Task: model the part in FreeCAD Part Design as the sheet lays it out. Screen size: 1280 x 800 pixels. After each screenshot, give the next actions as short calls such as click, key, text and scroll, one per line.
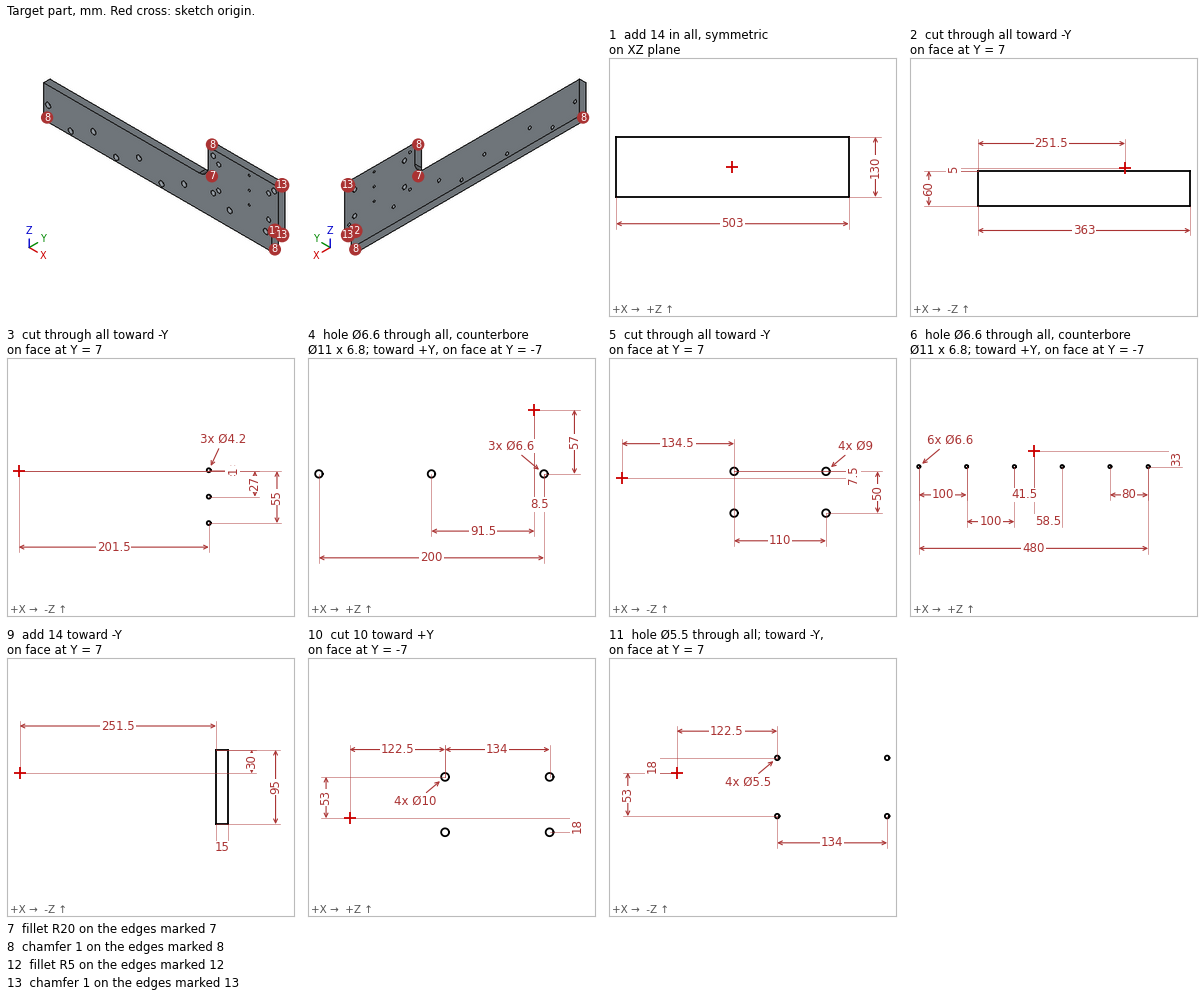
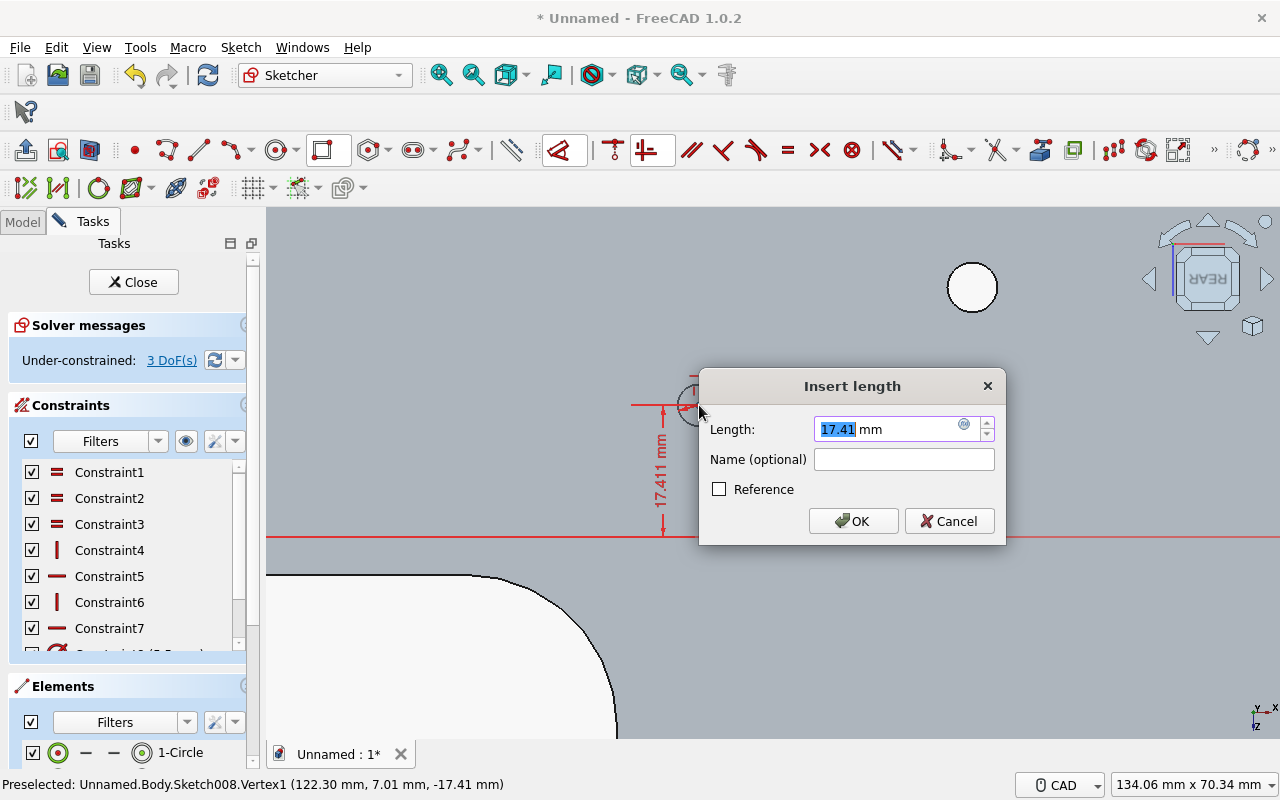
text(18)
key(Return)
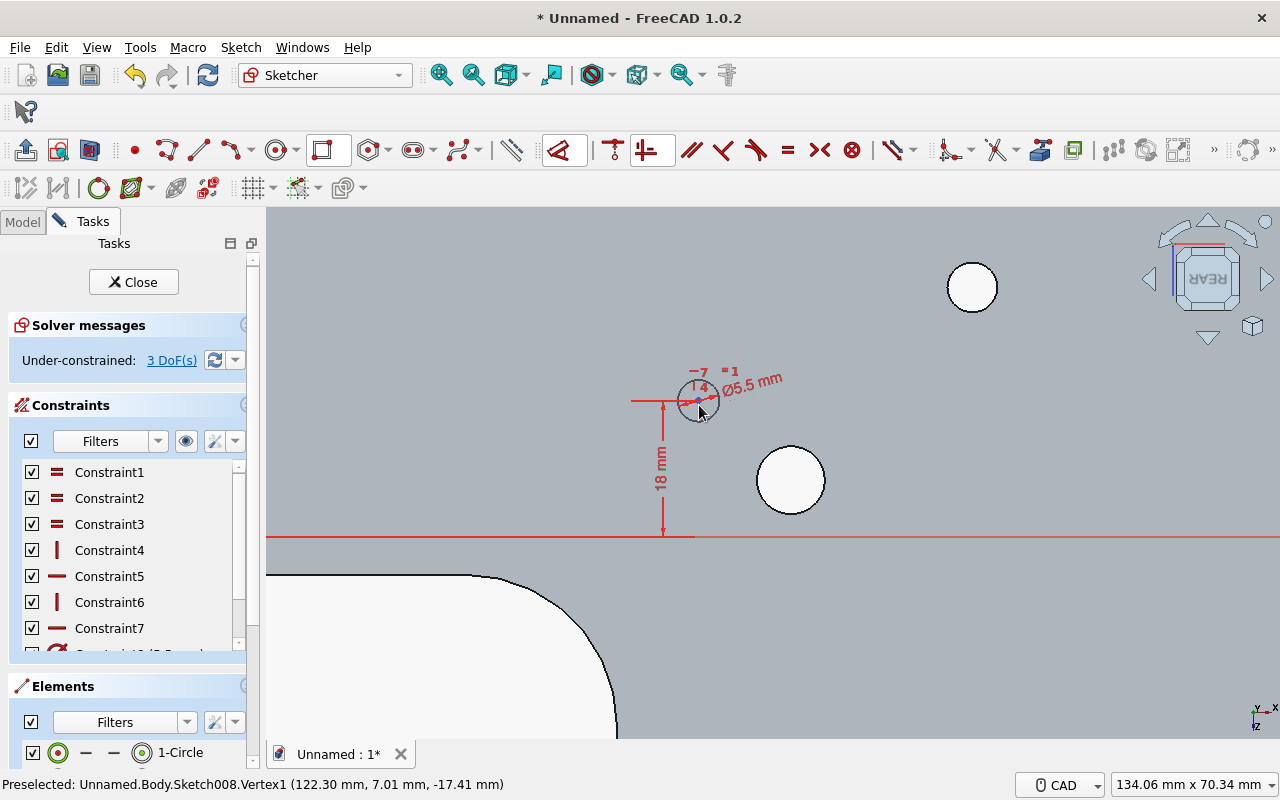
scroll(683, 388, down, 6)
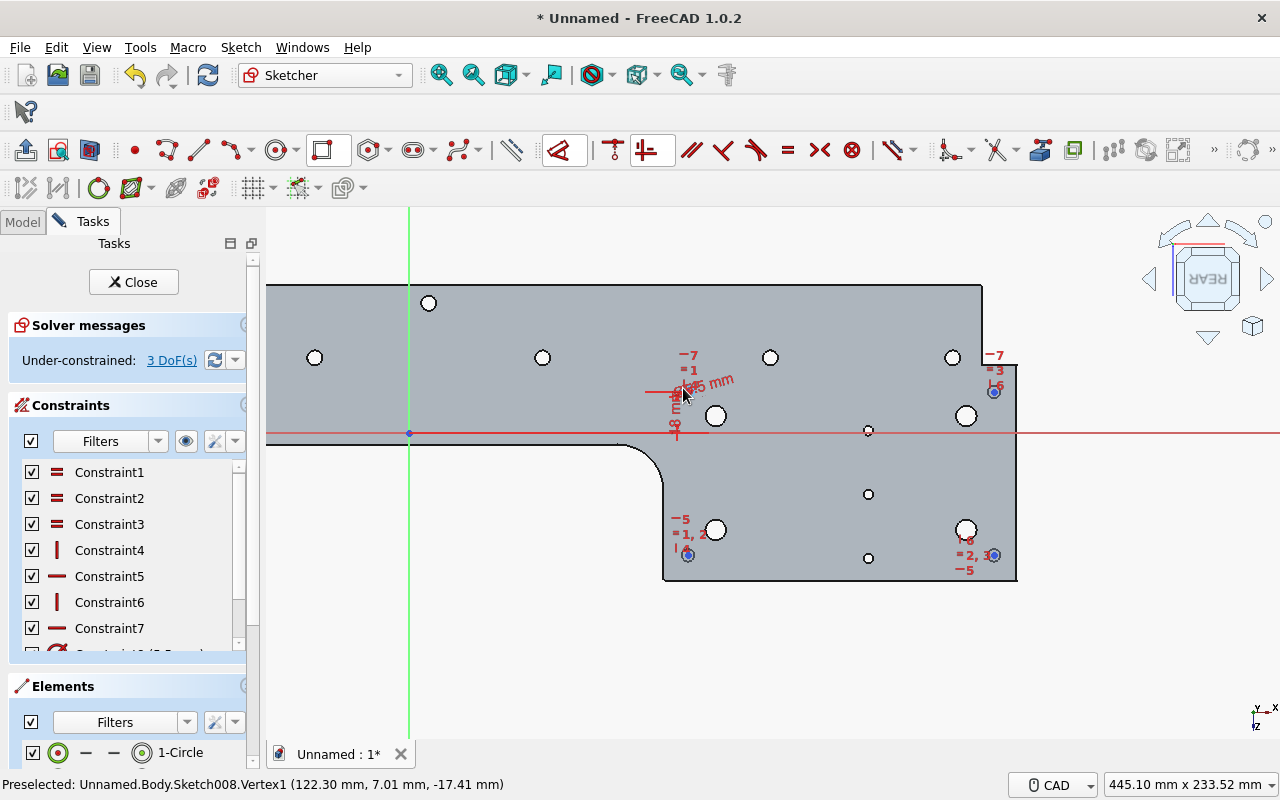
click(688, 555)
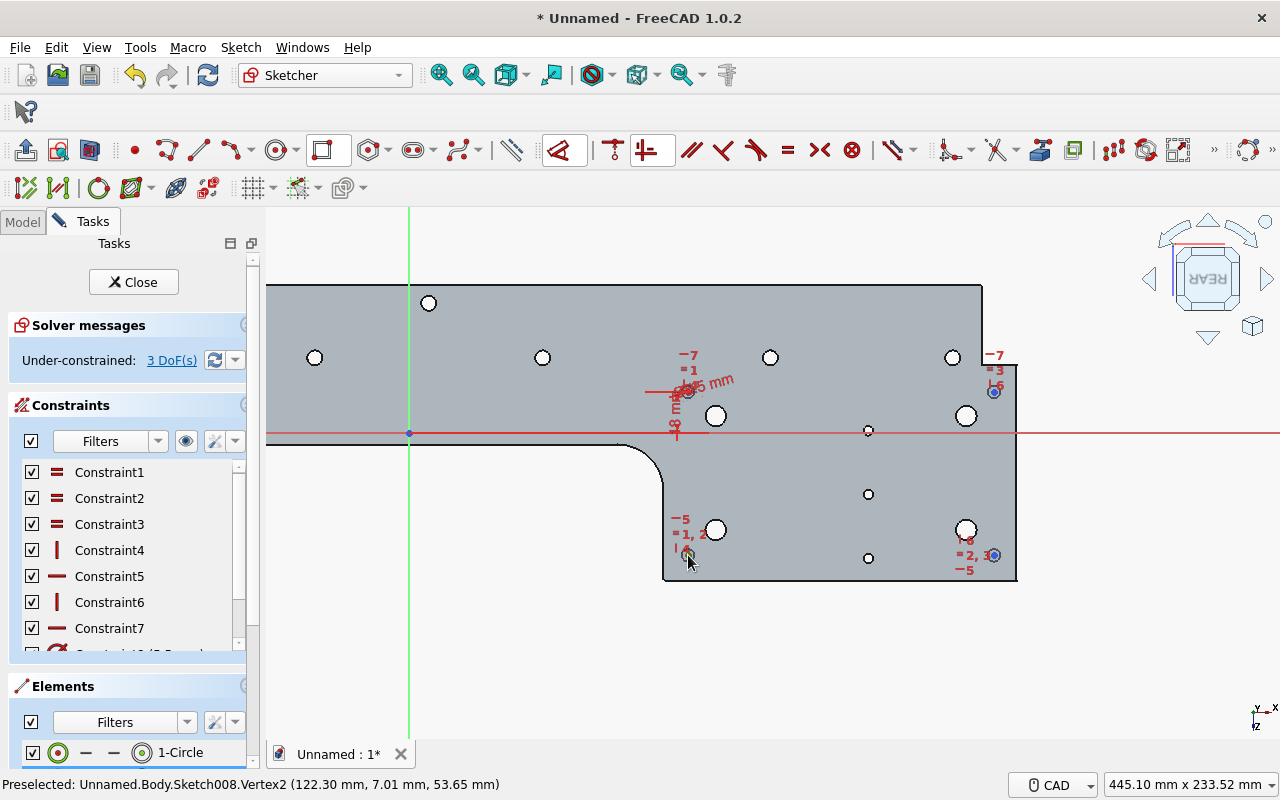
key(i)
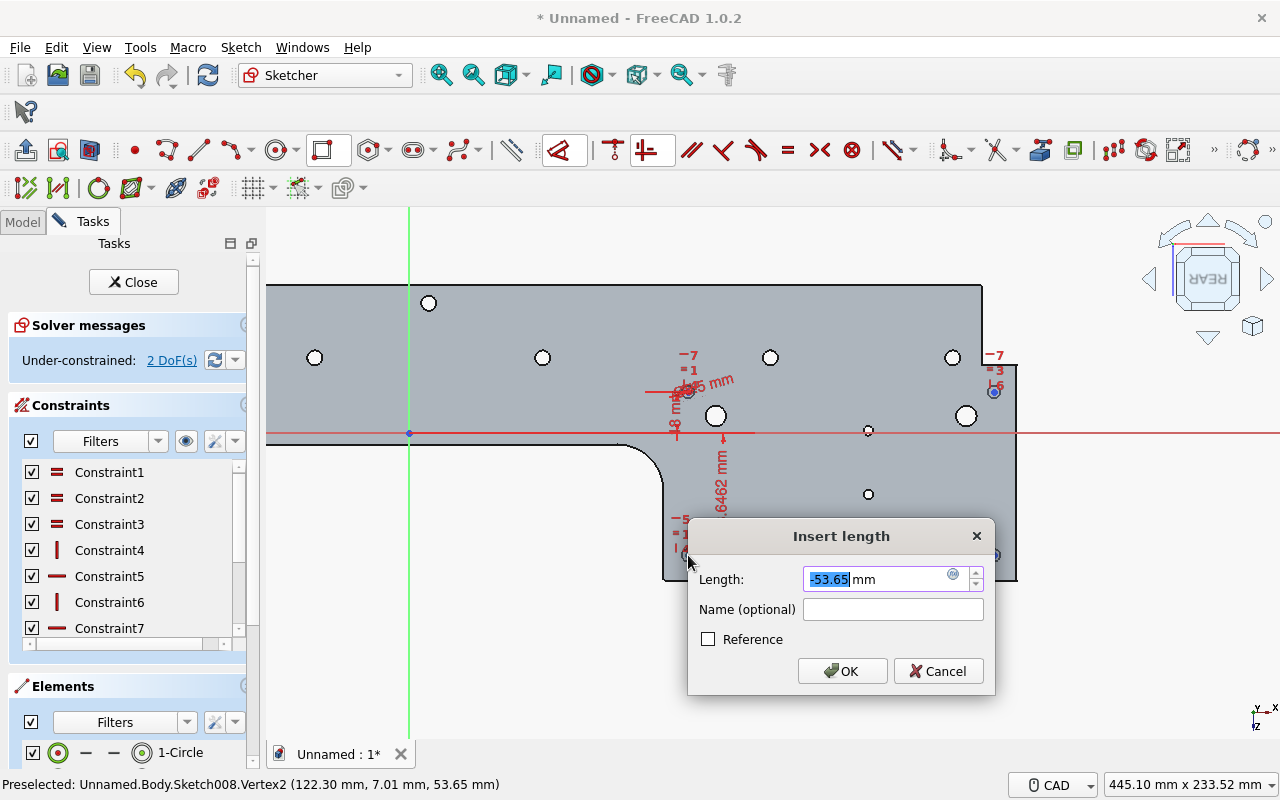
text(-53)
key(Return)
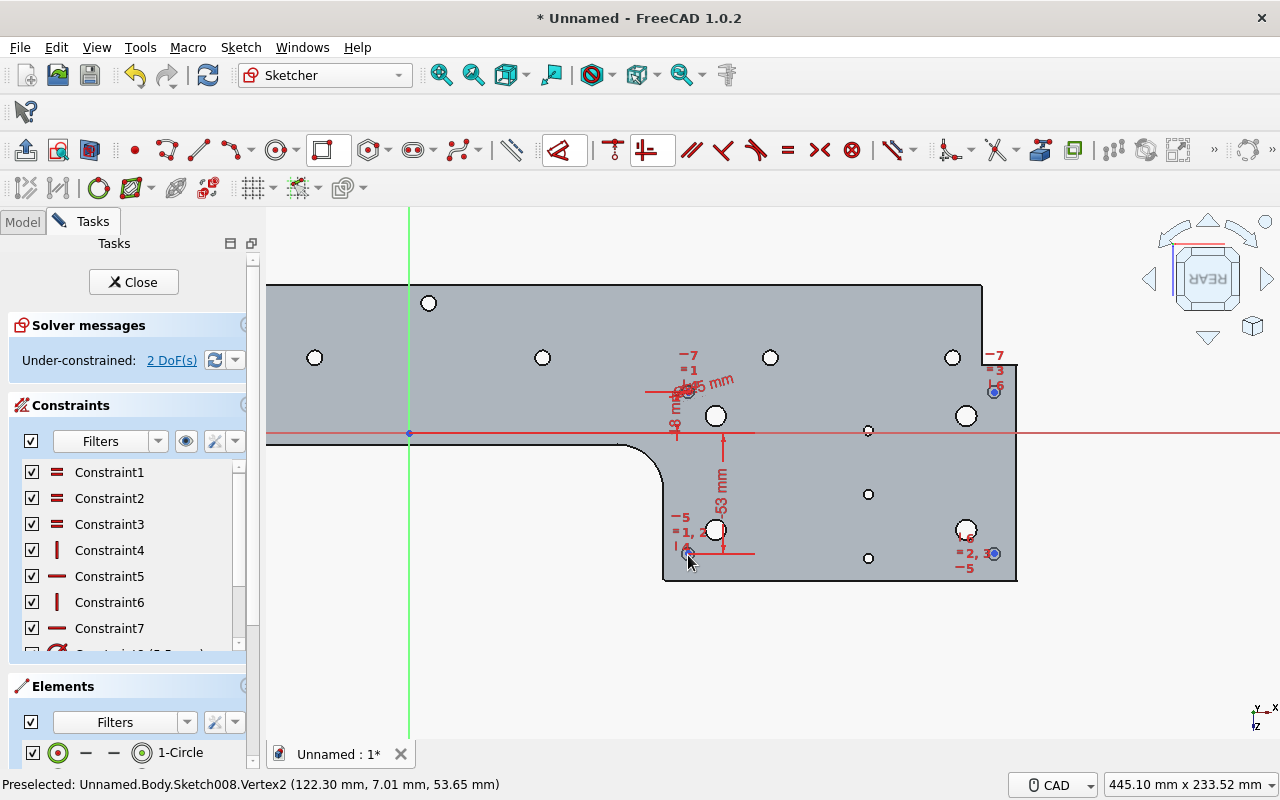
click(688, 554)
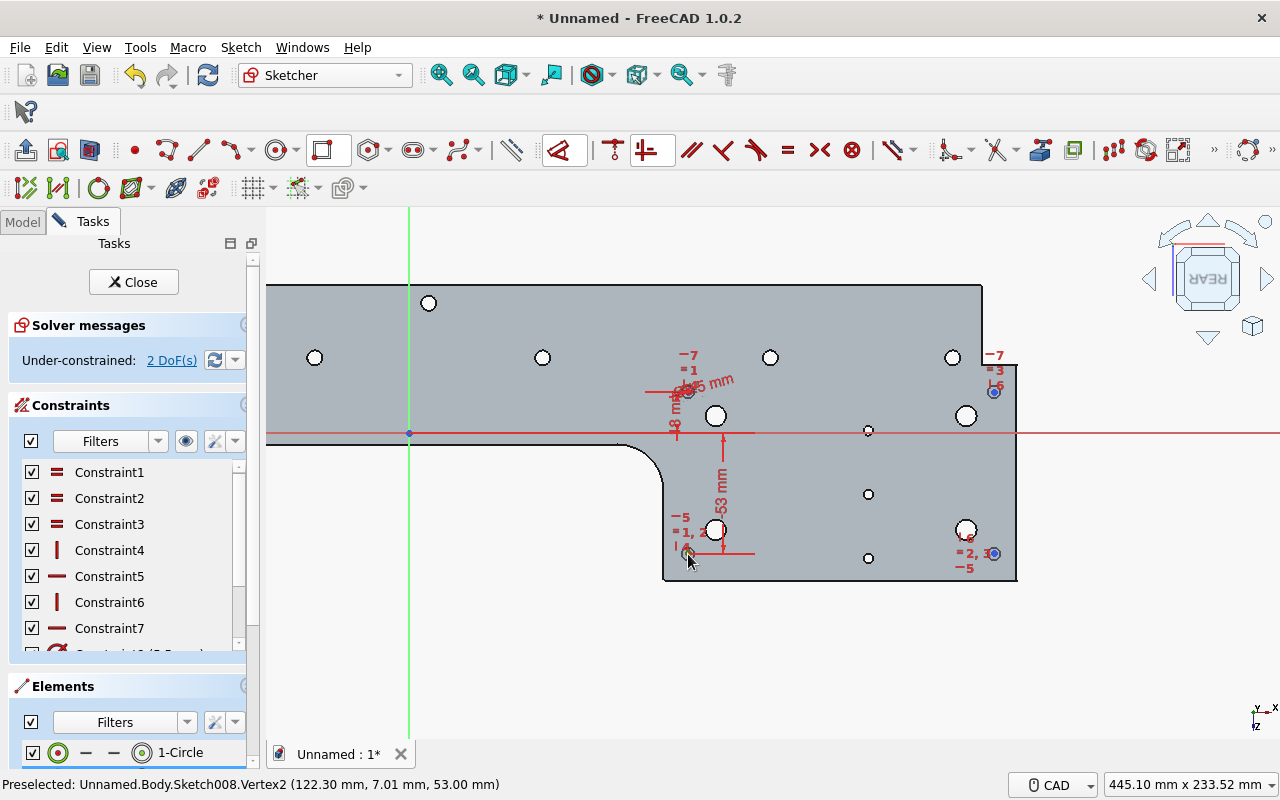
click(994, 554)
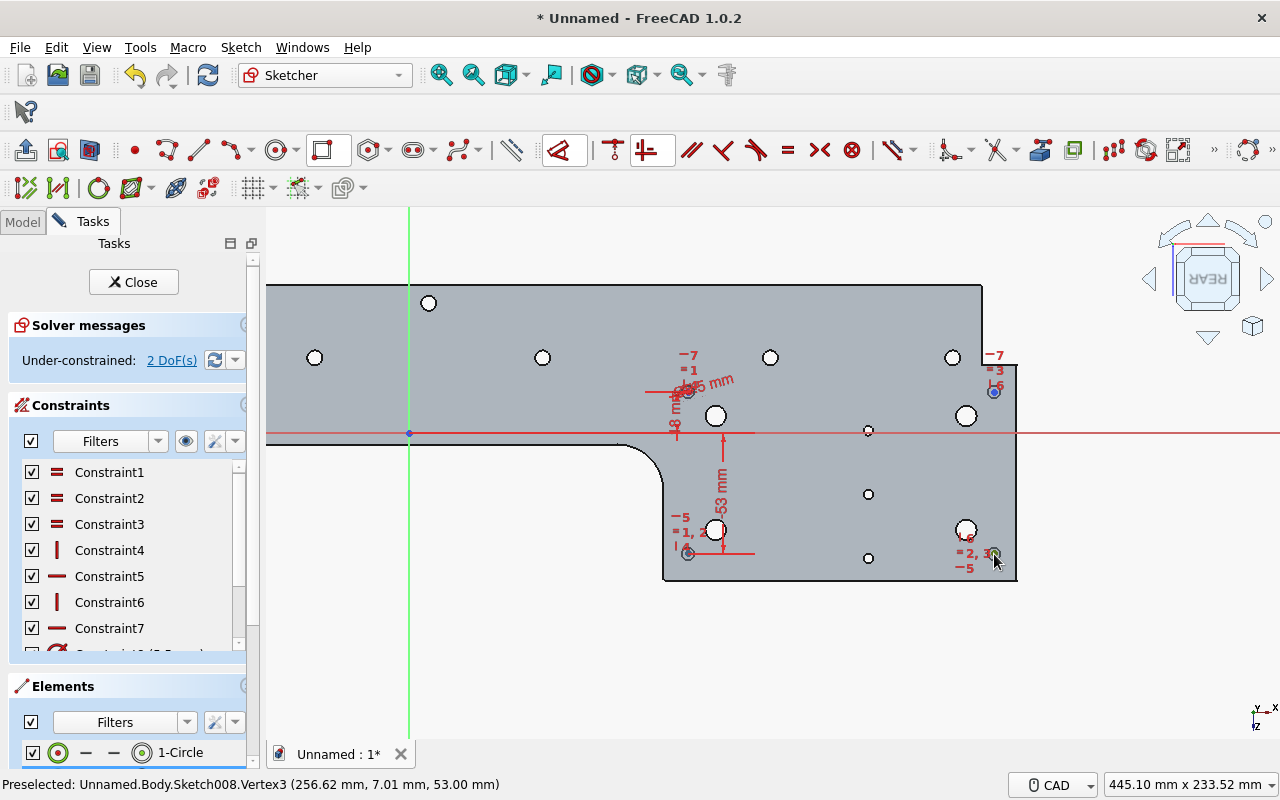
key(l)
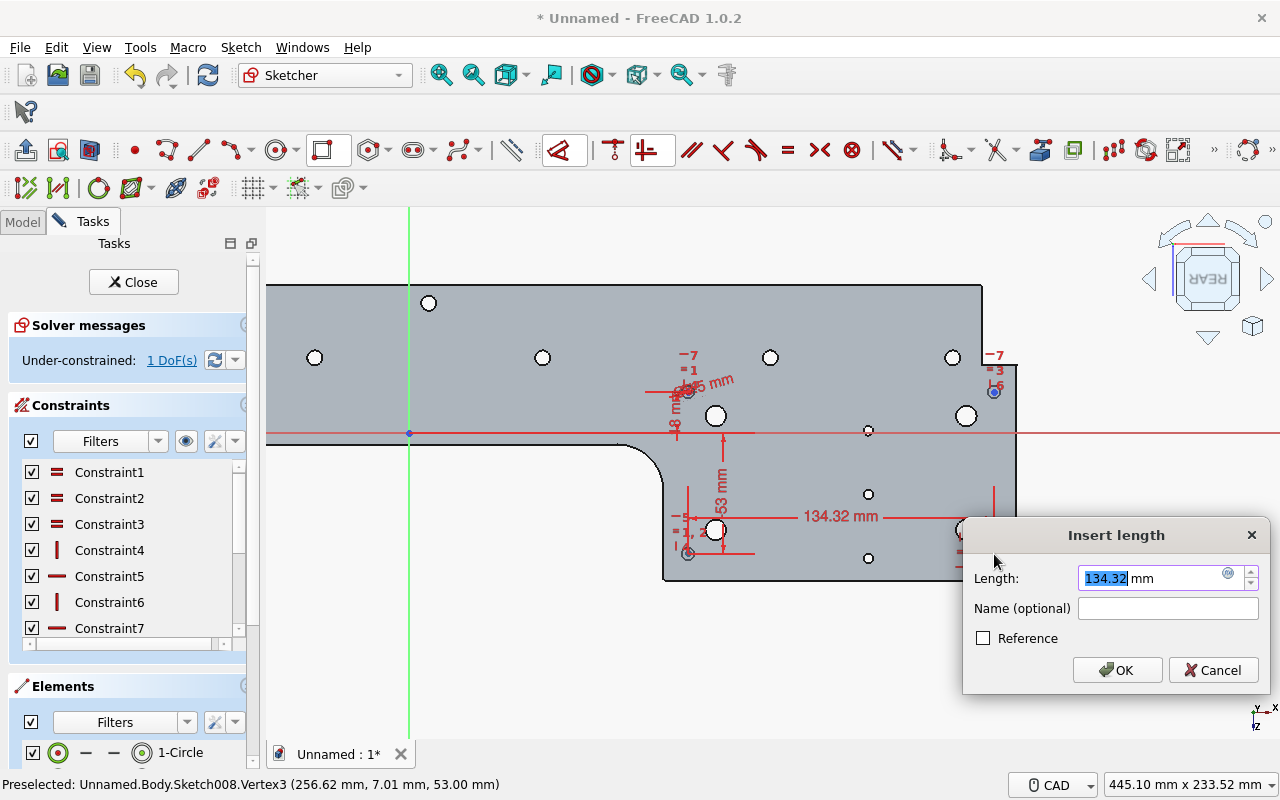
text(134)
key(Return)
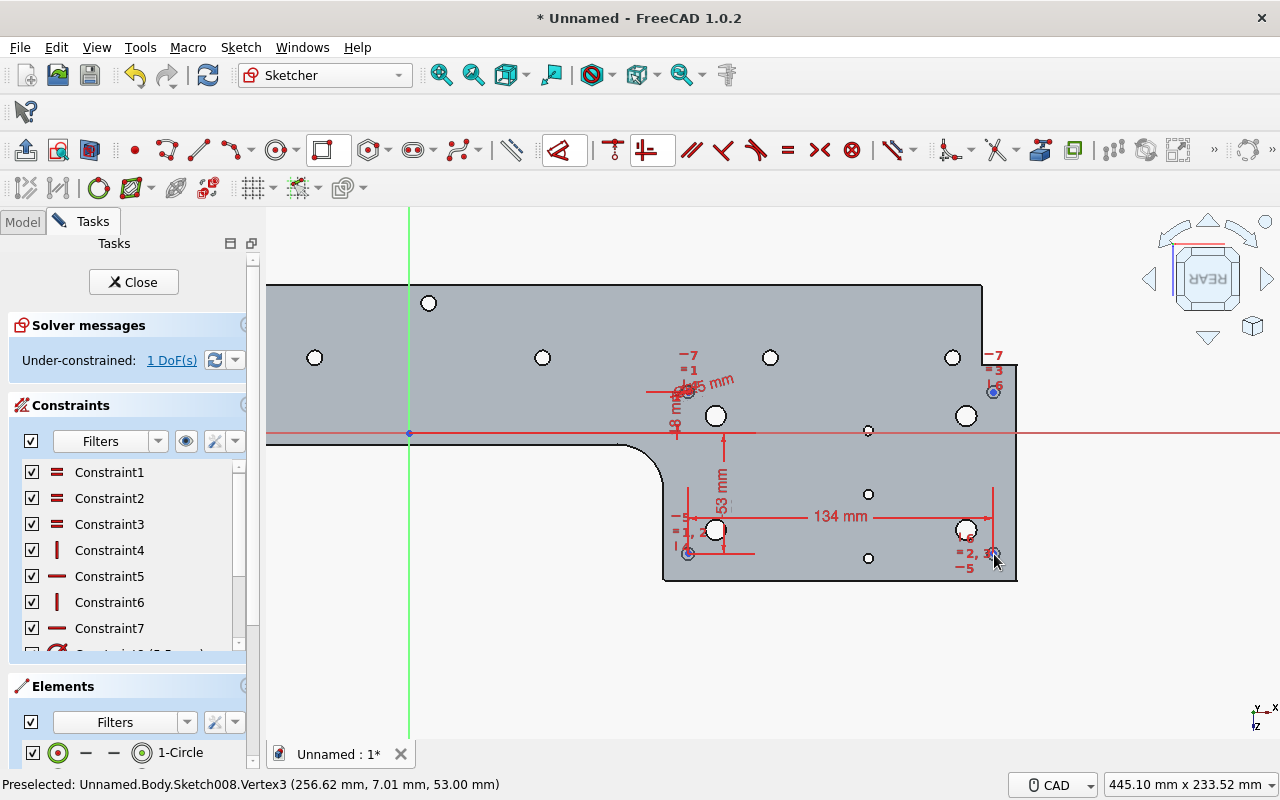
click(688, 392)